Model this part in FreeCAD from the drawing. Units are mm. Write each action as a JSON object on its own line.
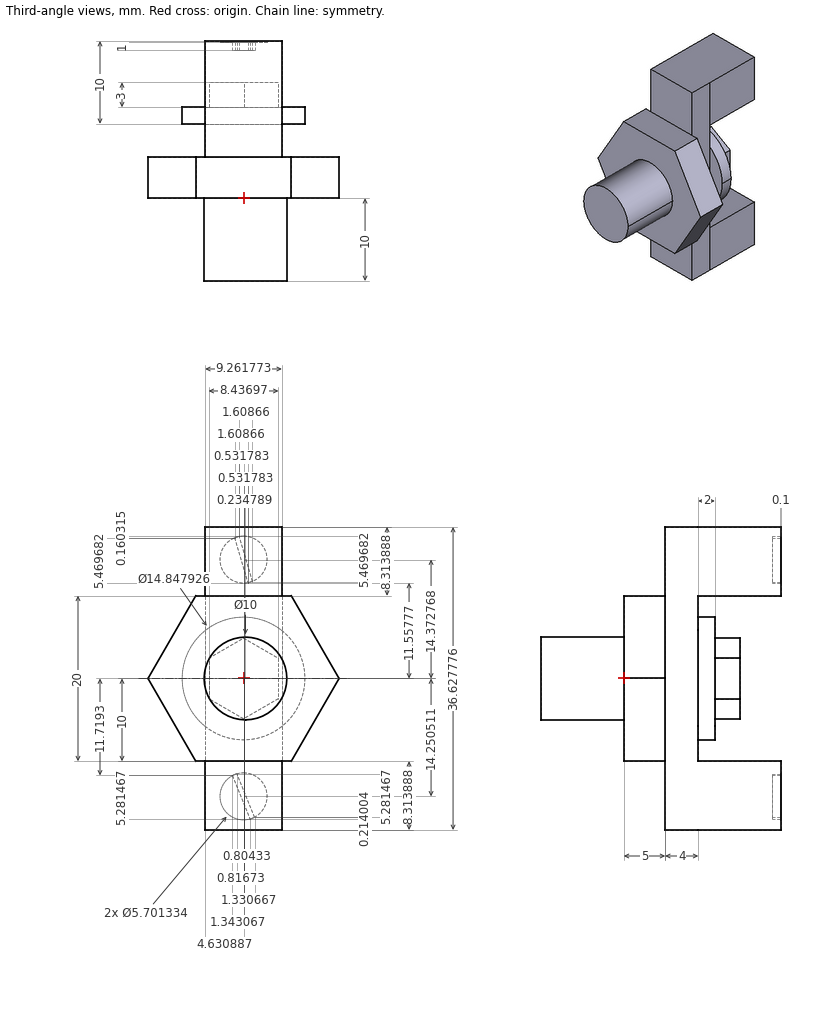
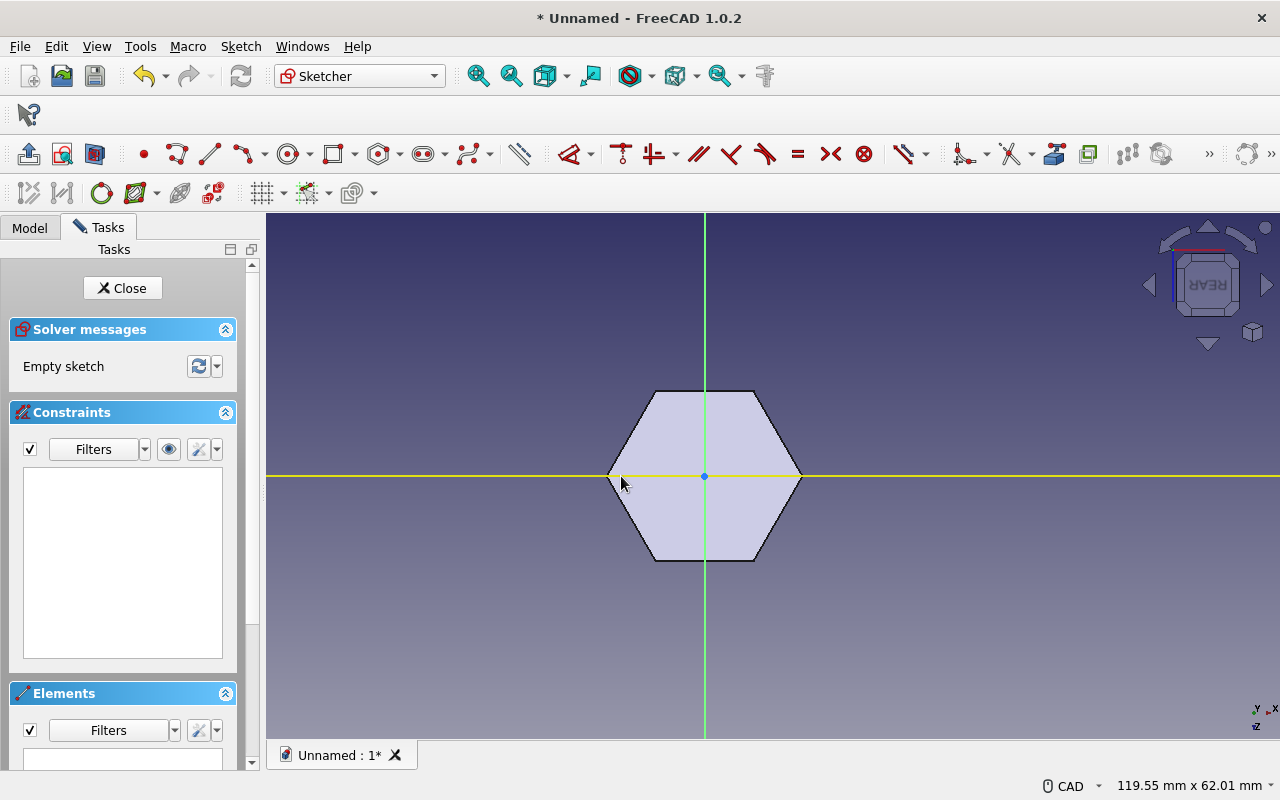
{"action": "left_click", "coordinate": [354, 154]}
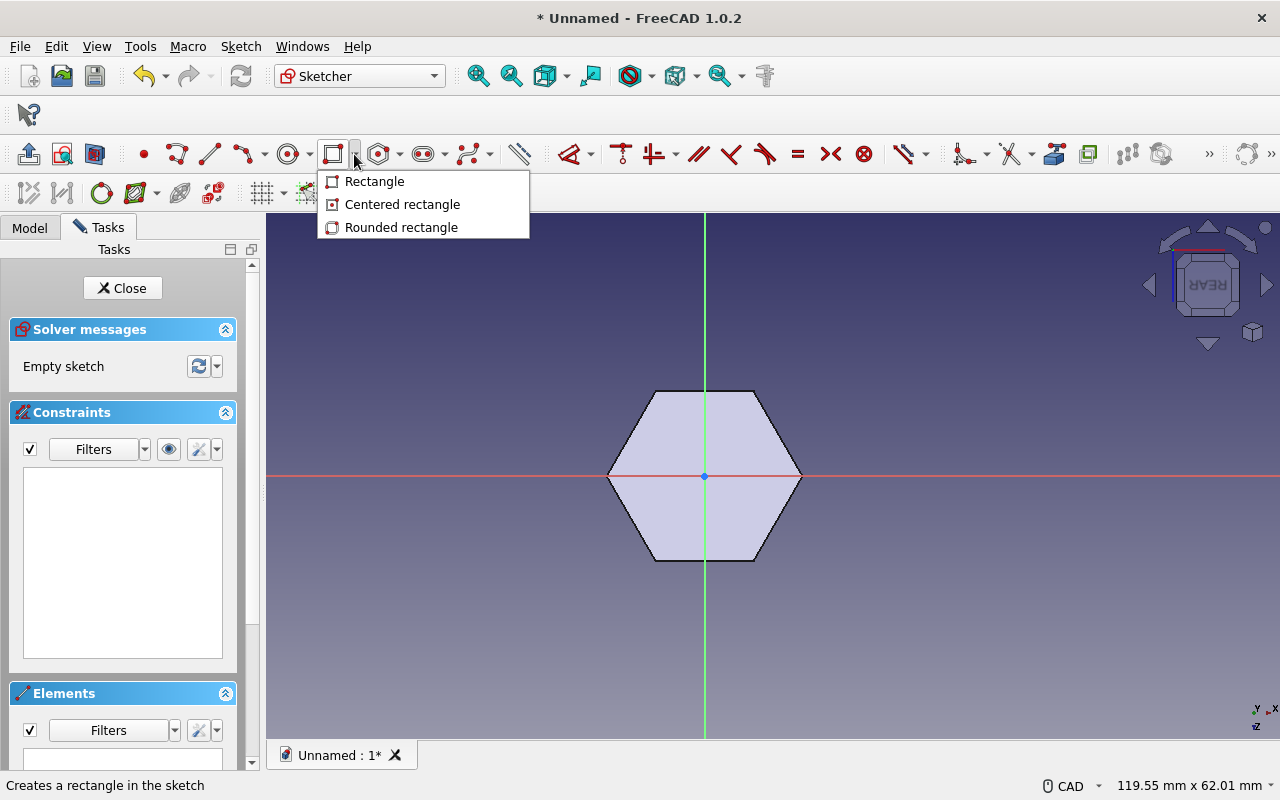
{"action": "left_click", "coordinate": [424, 204]}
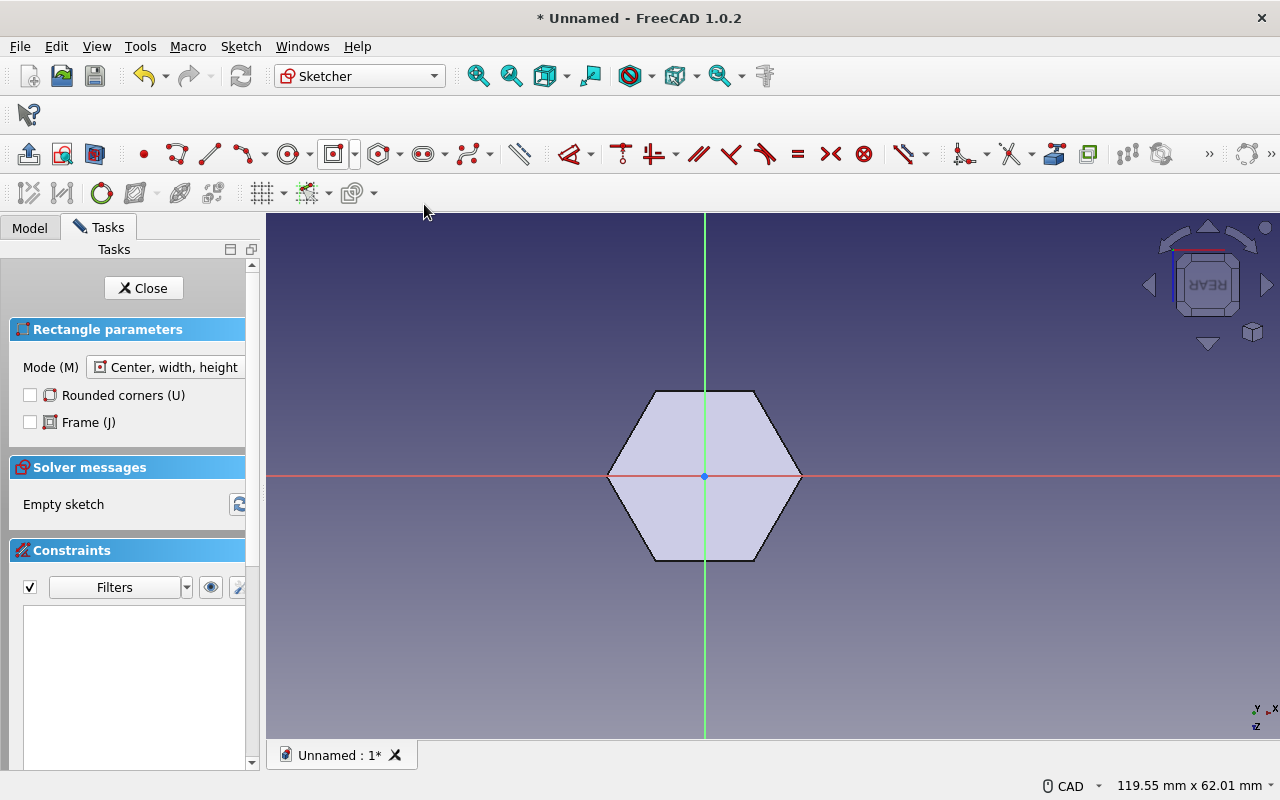
{"action": "left_click", "coordinate": [705, 476]}
{"action": "mouse_move", "coordinate": [744, 321]}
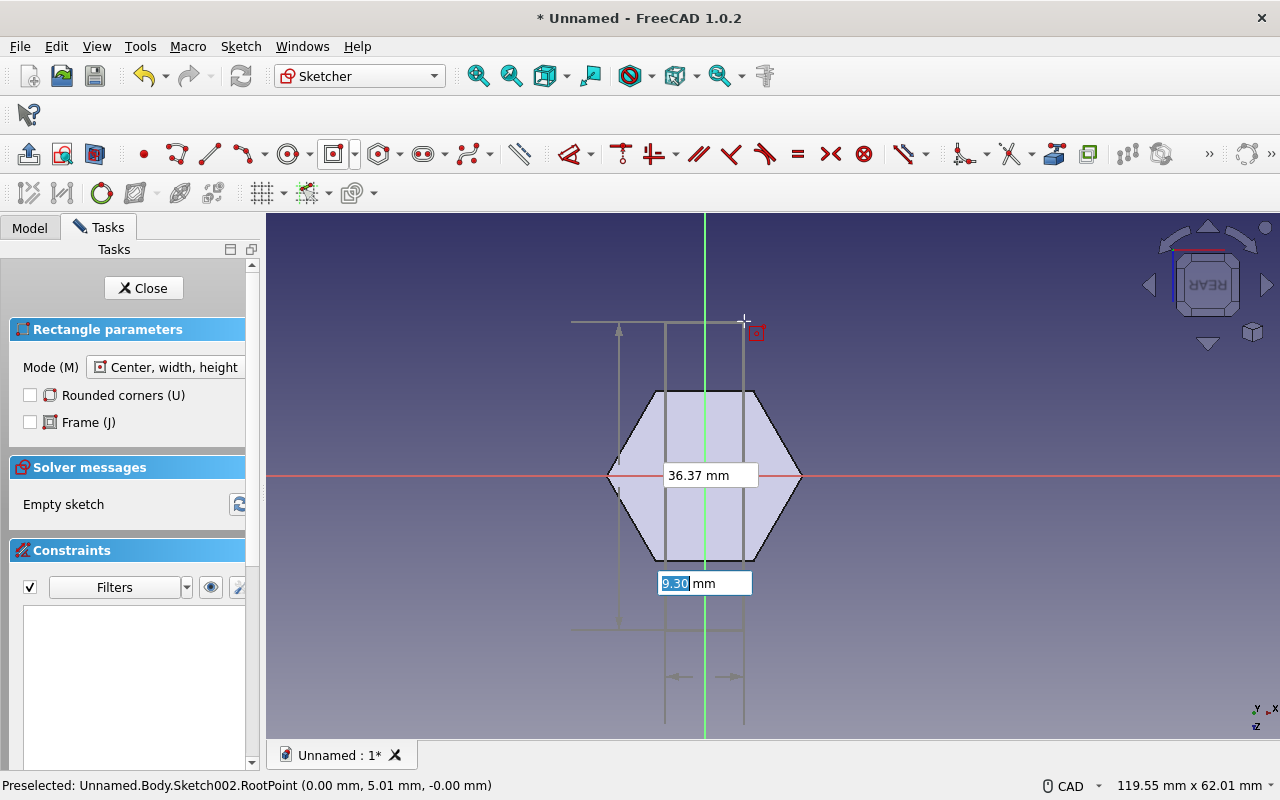
{"action": "type", "text": "9.261773"}
{"action": "key", "text": "Tab"}
{"action": "type", "text": "36.627776"}
{"action": "key", "text": "Return"}
{"action": "key", "text": "Escape"}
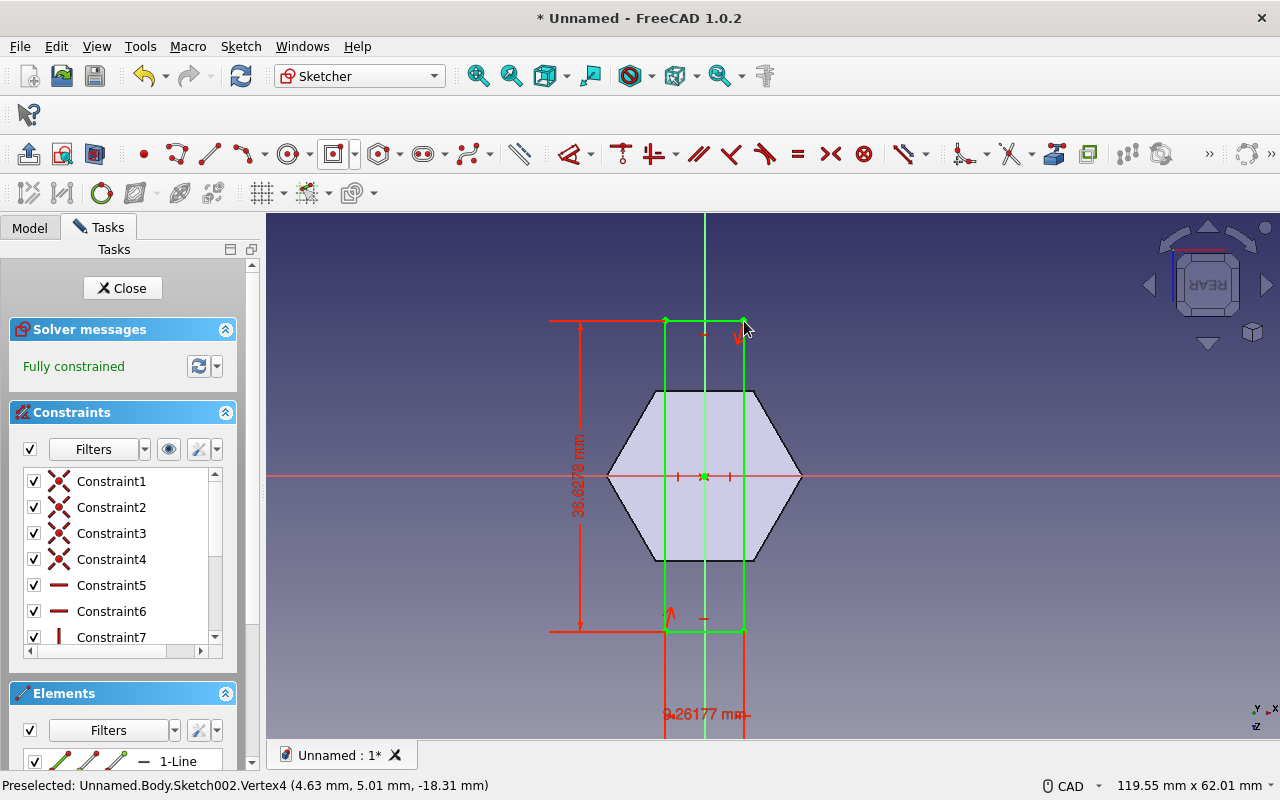
{"action": "left_click", "coordinate": [123, 288]}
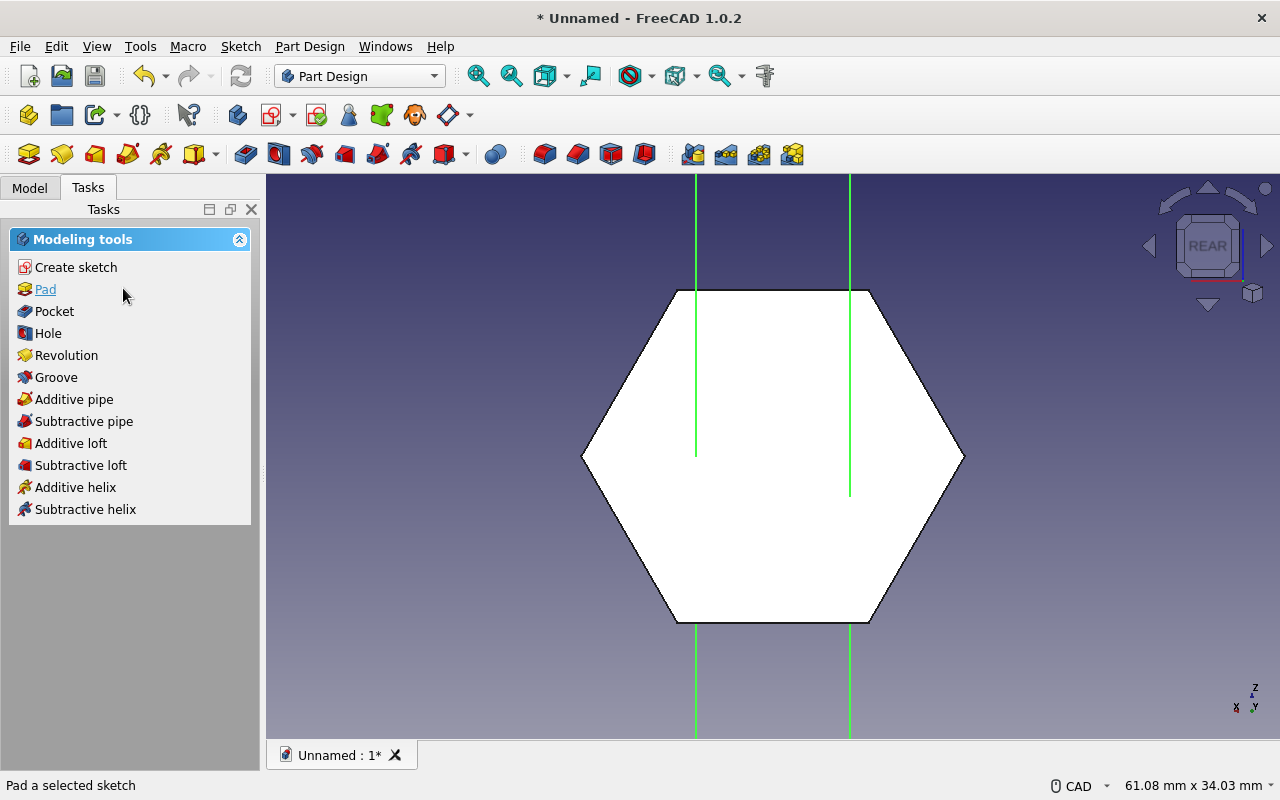
{"action": "left_click", "coordinate": [29, 154]}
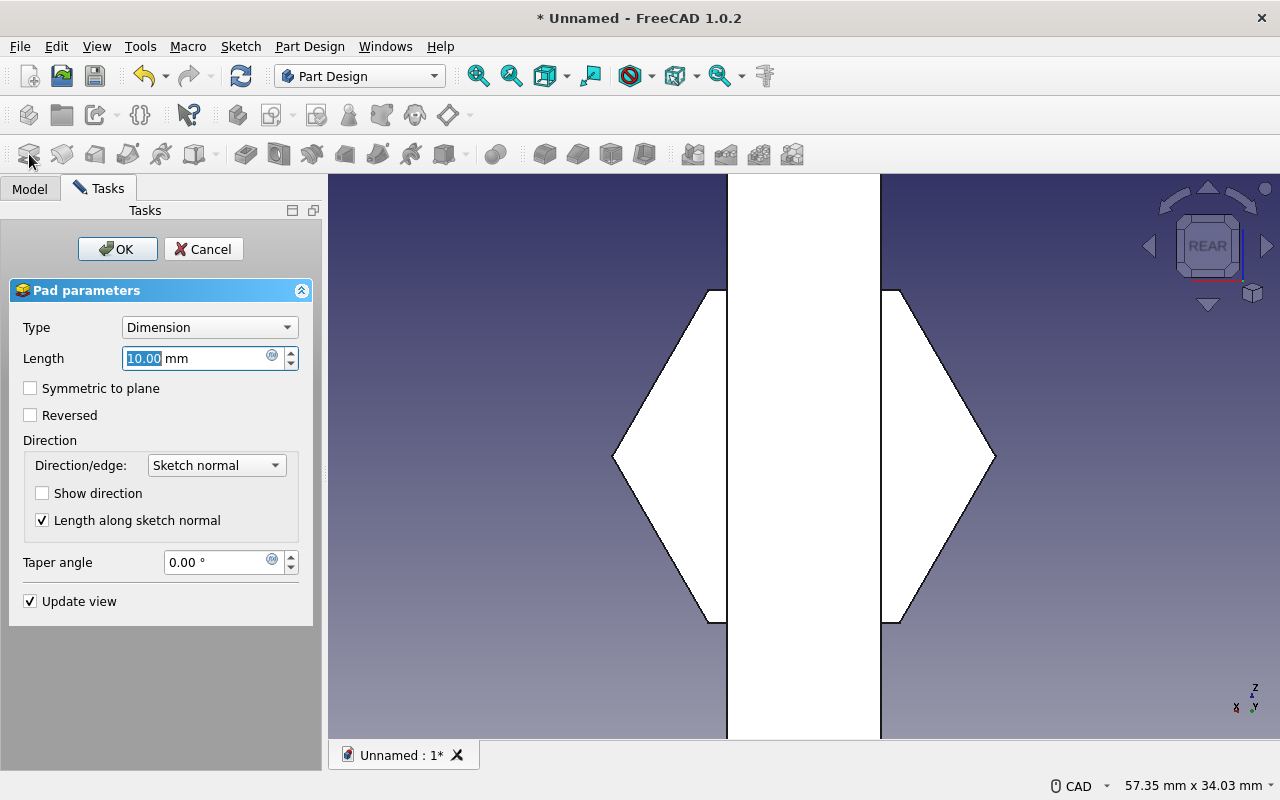
{"action": "type", "text": "4"}
{"action": "key", "text": "Tab"}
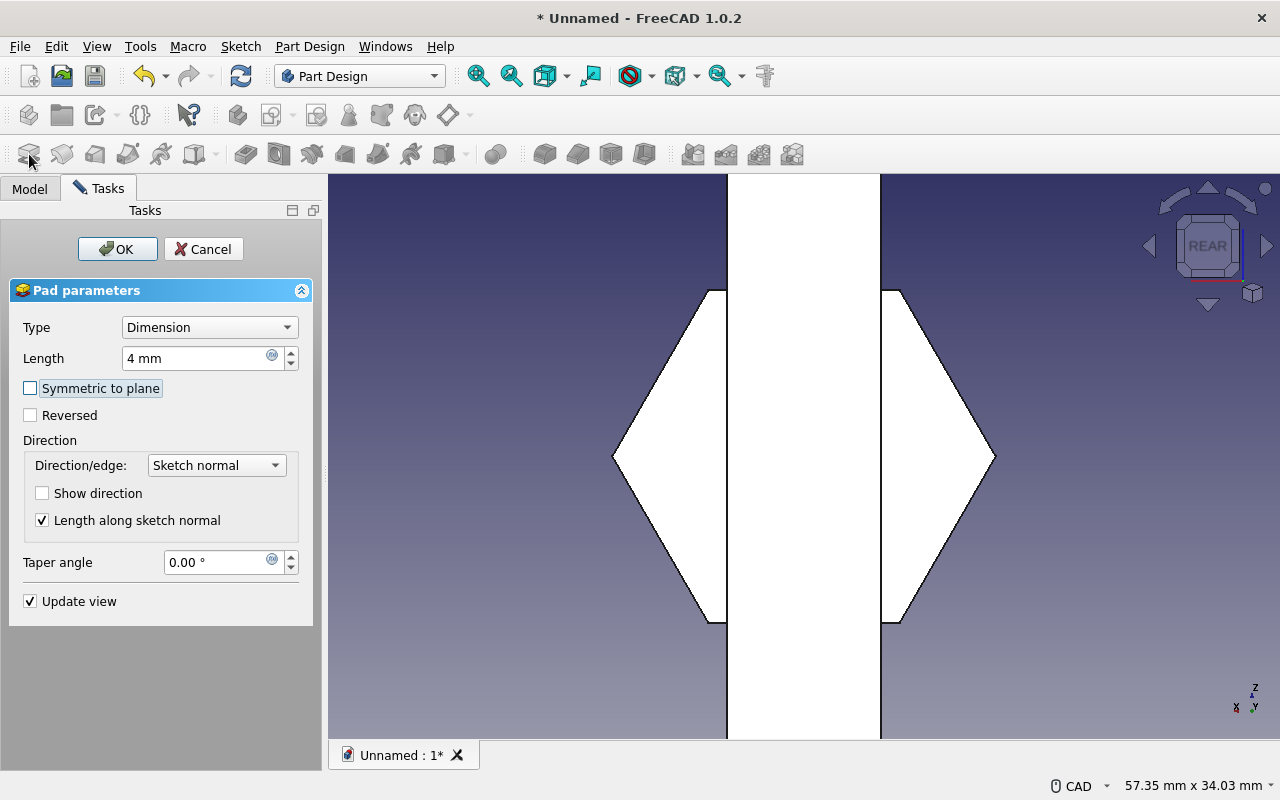
{"action": "left_click", "coordinate": [118, 249]}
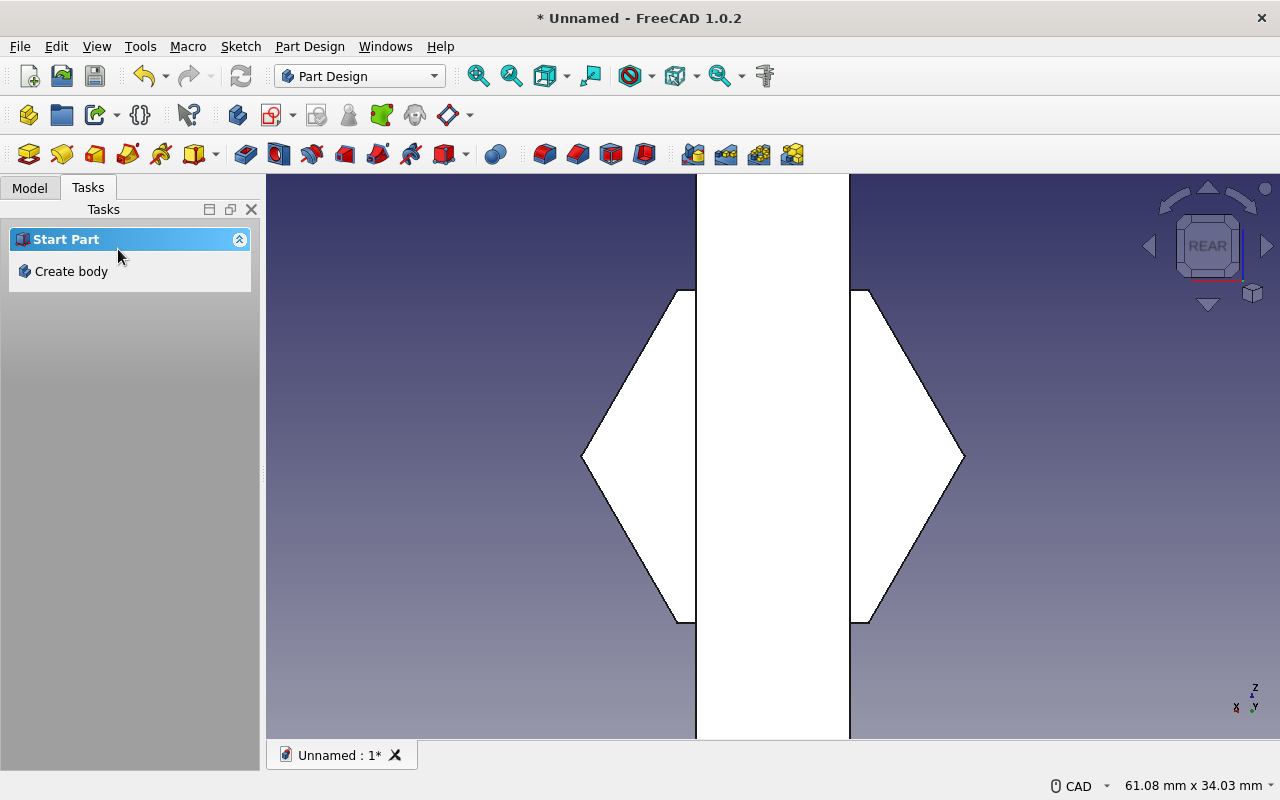
{"action": "left_click", "coordinate": [479, 76]}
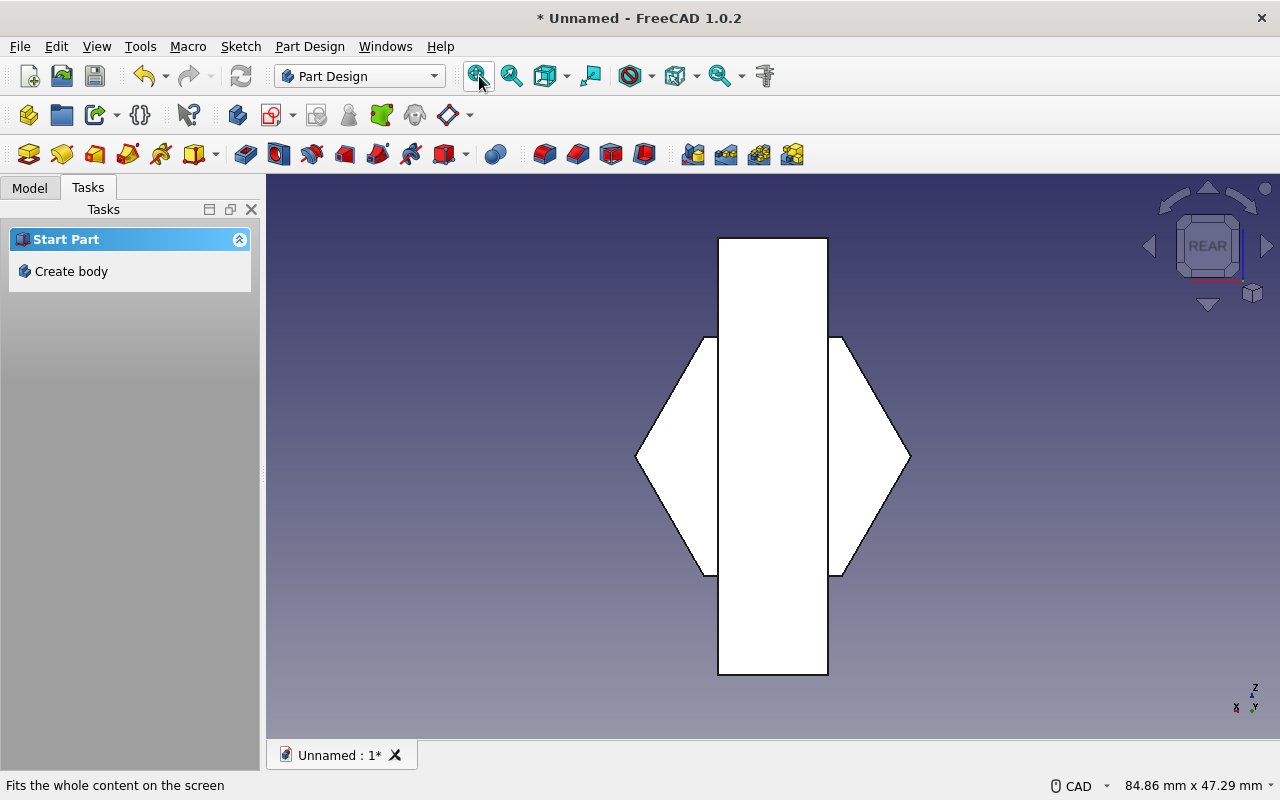
{"action": "left_click", "coordinate": [773, 581]}